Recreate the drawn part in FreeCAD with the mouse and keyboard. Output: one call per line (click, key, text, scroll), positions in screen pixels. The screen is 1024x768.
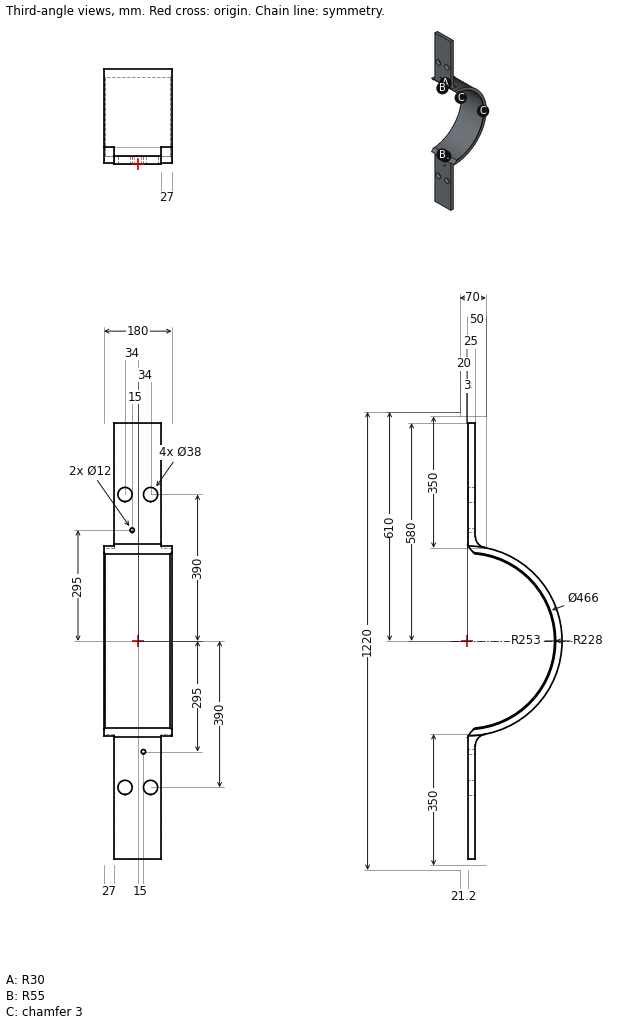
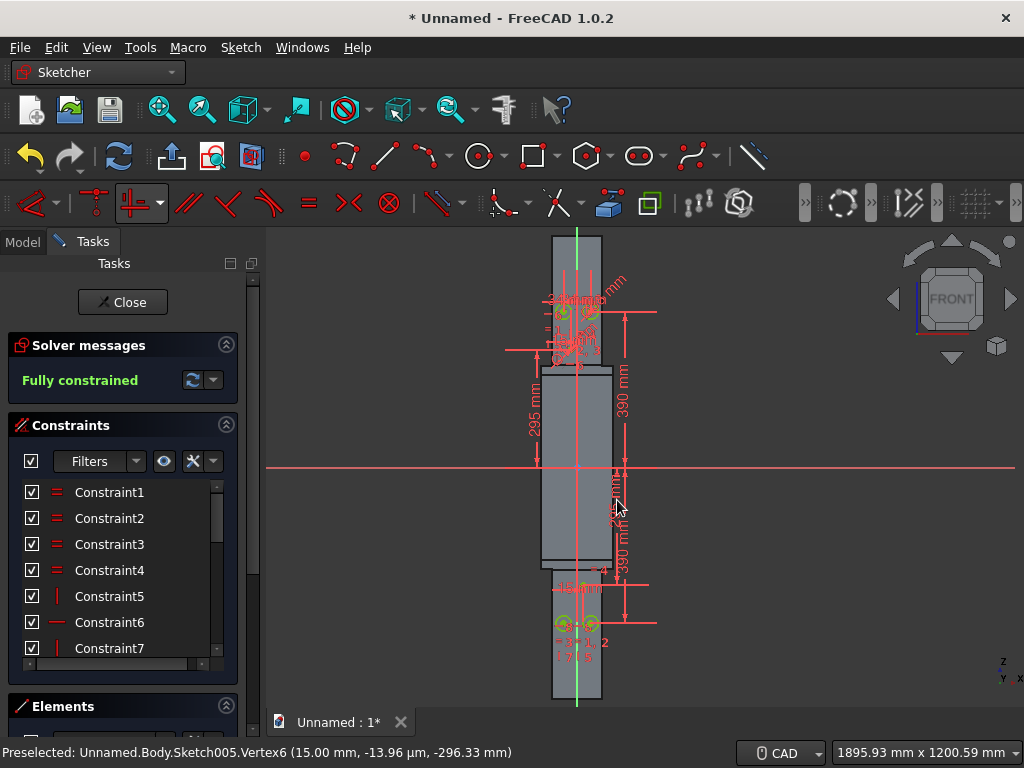
click(123, 302)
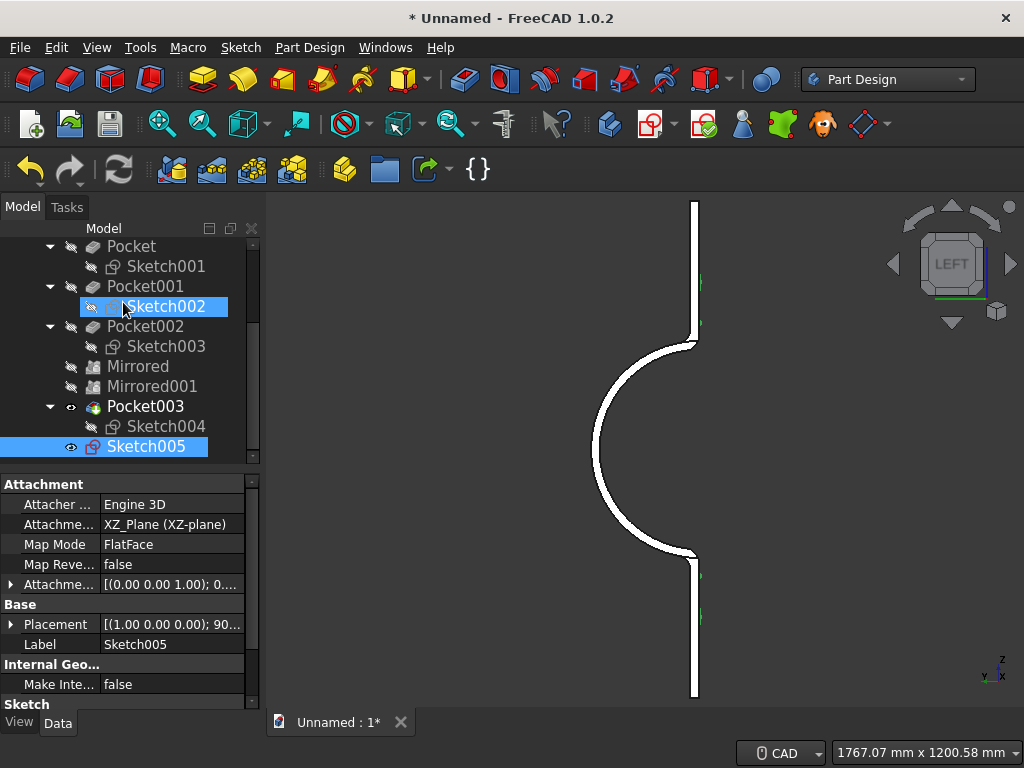
click(466, 80)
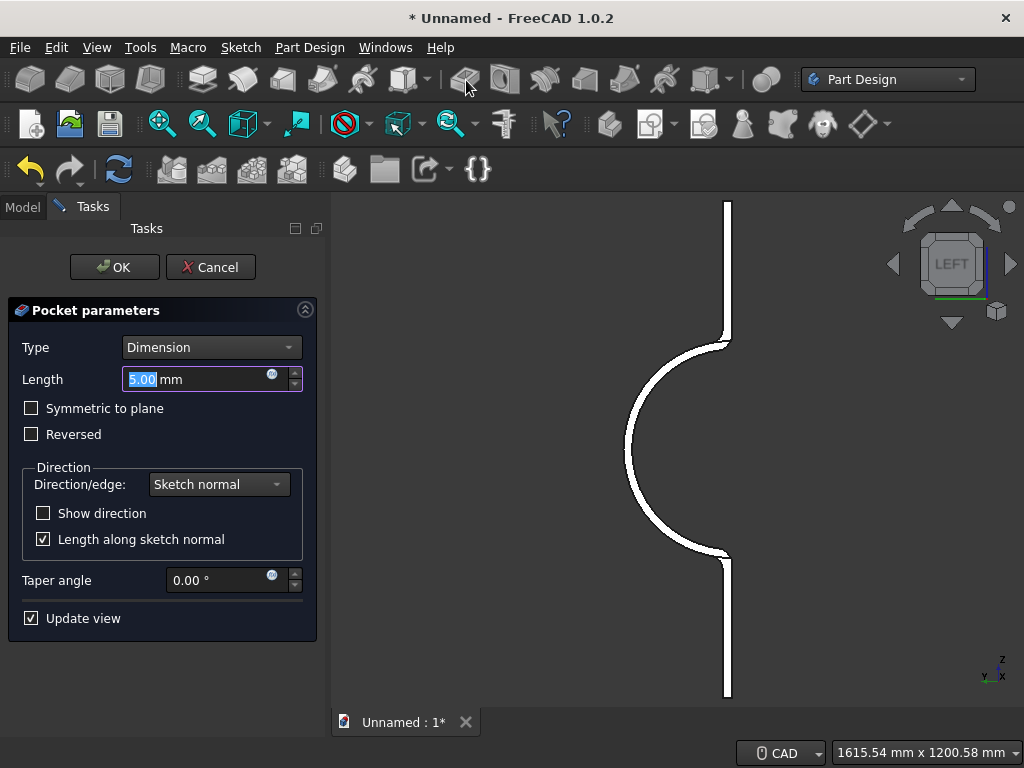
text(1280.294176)
key(Tab)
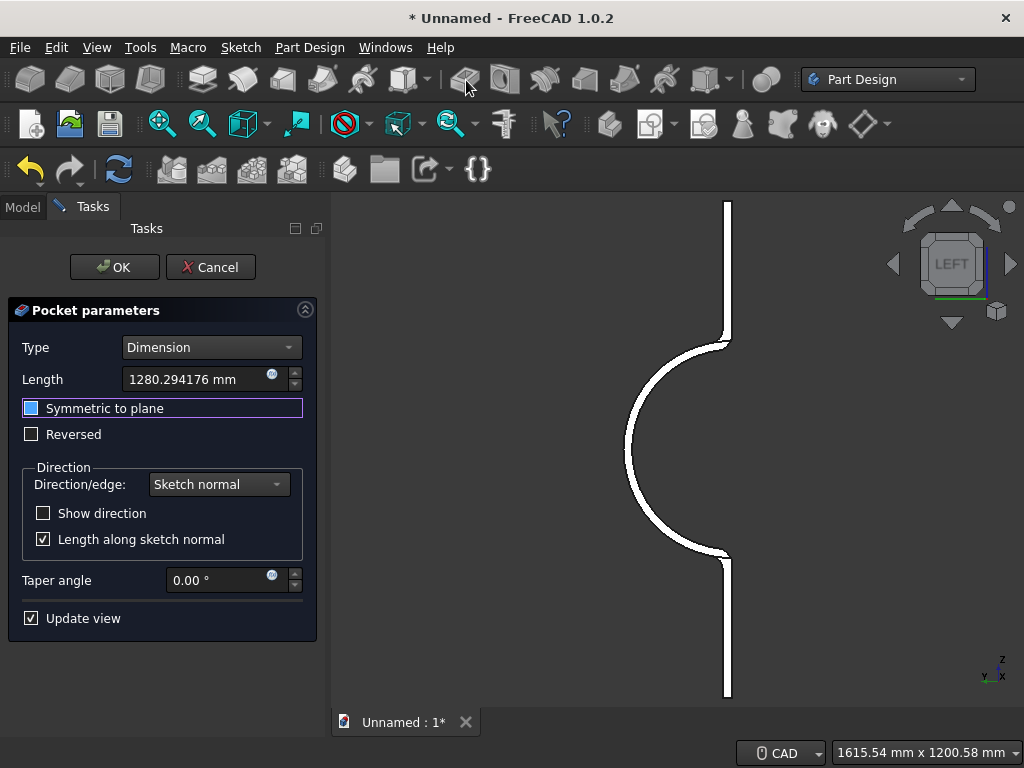
click(30, 408)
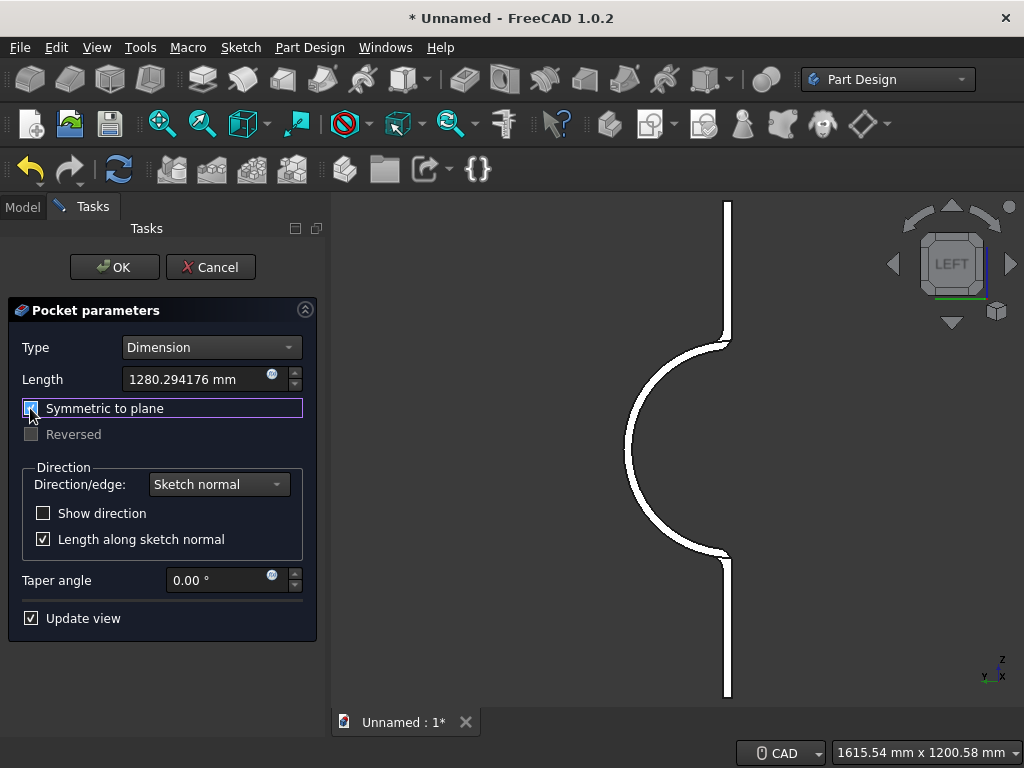
click(115, 267)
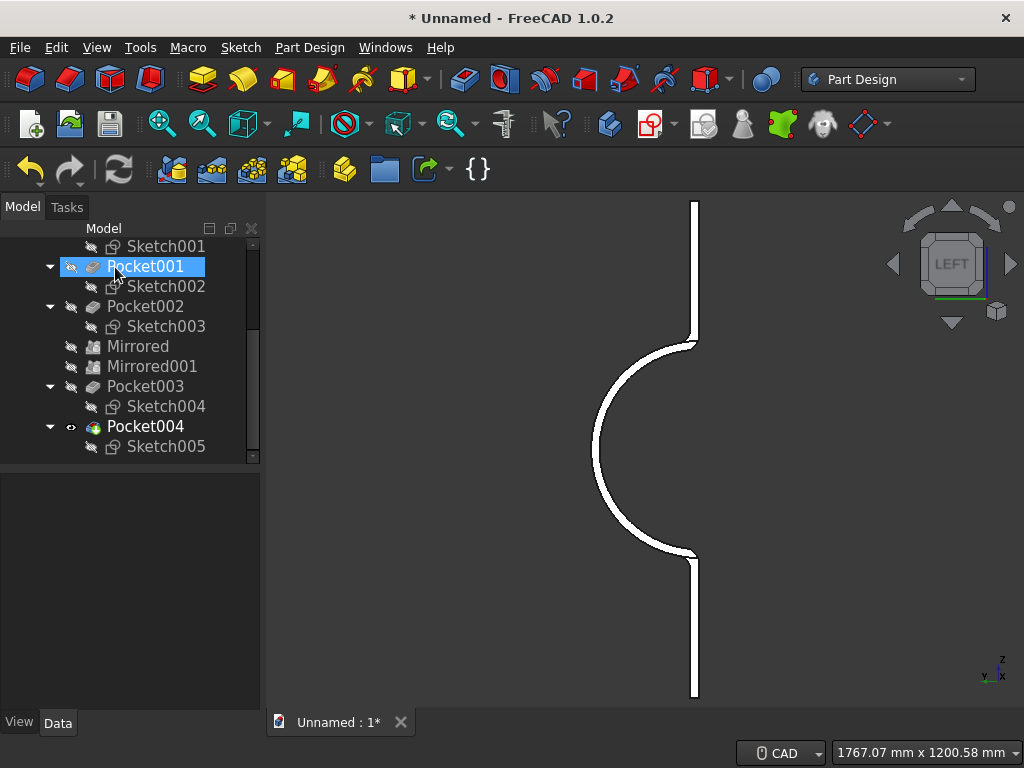
click(626, 516)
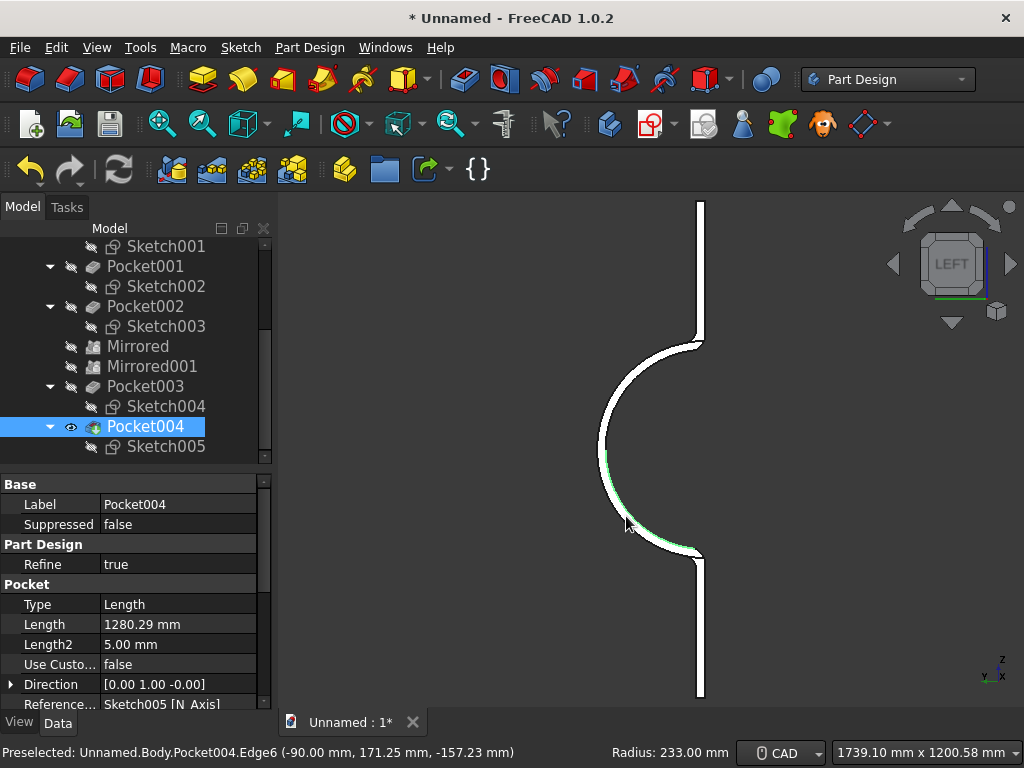
key(0)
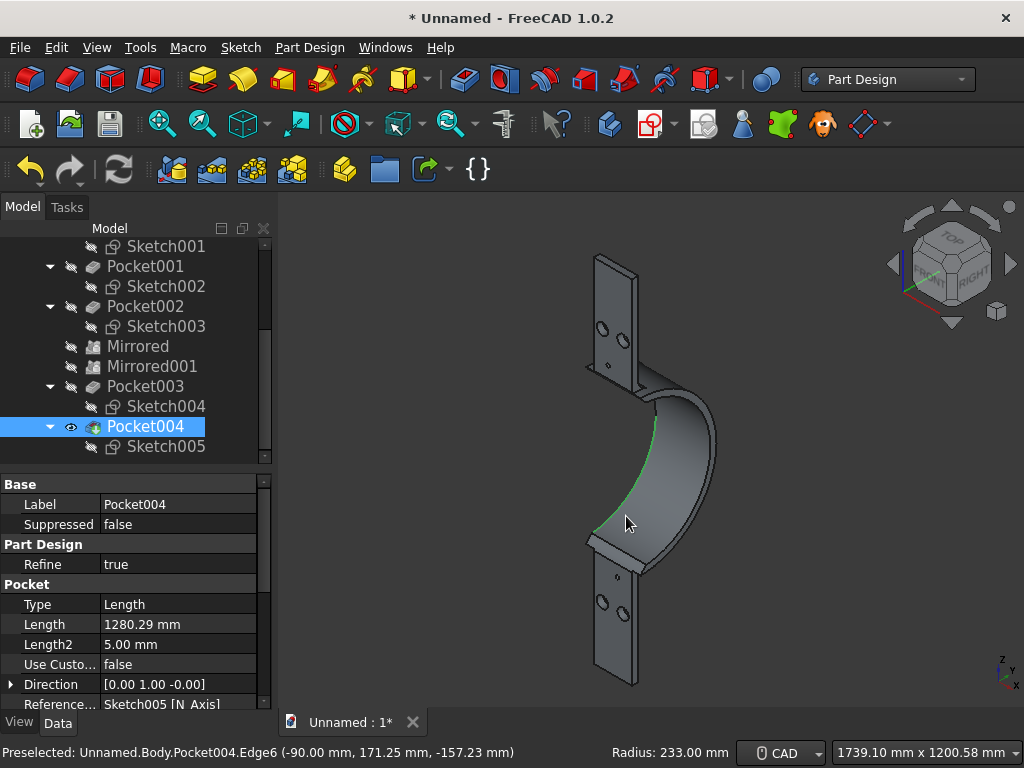
click(692, 401, ctrl)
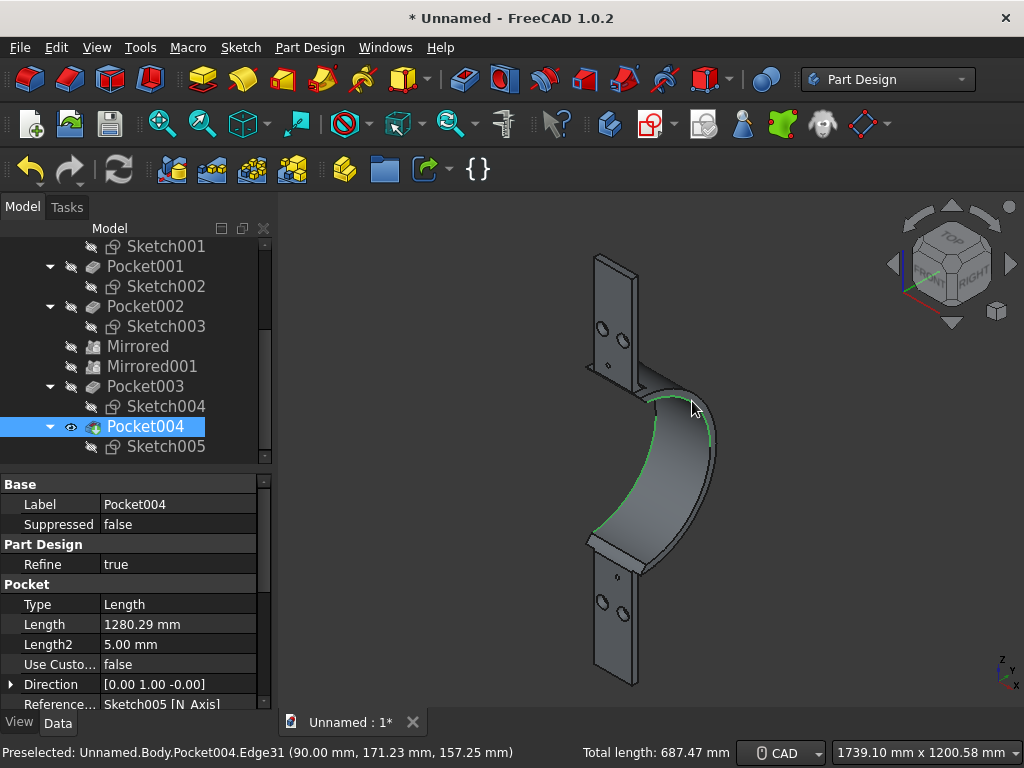
click(70, 80)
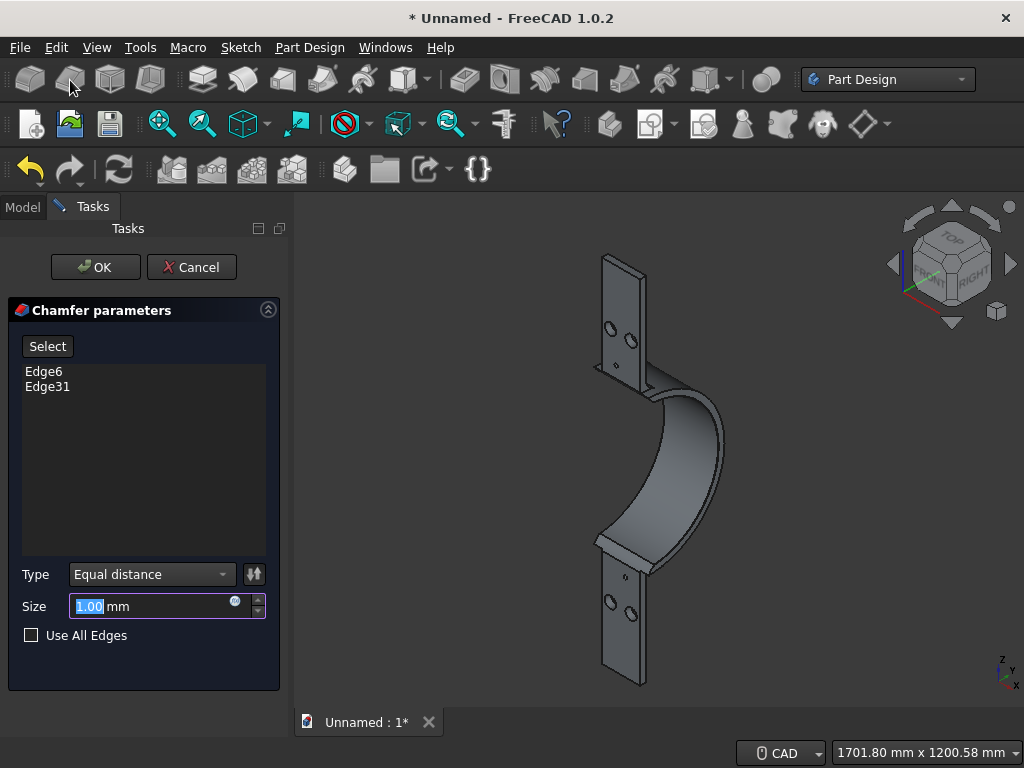
text(3)
key(Tab)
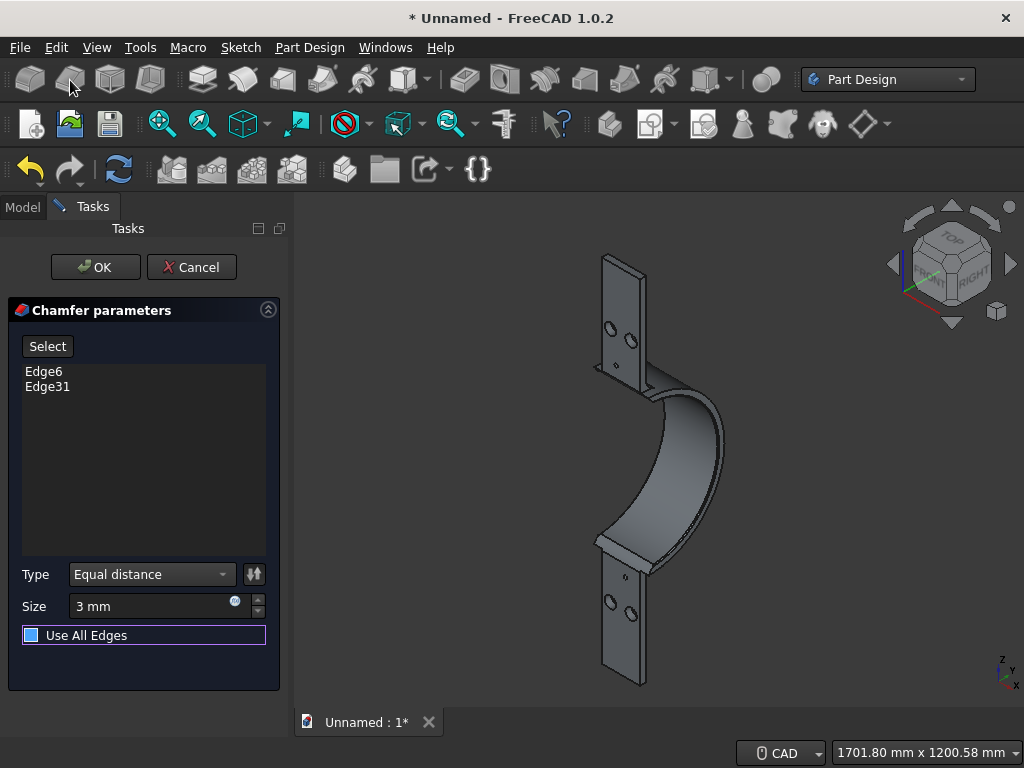
click(96, 267)